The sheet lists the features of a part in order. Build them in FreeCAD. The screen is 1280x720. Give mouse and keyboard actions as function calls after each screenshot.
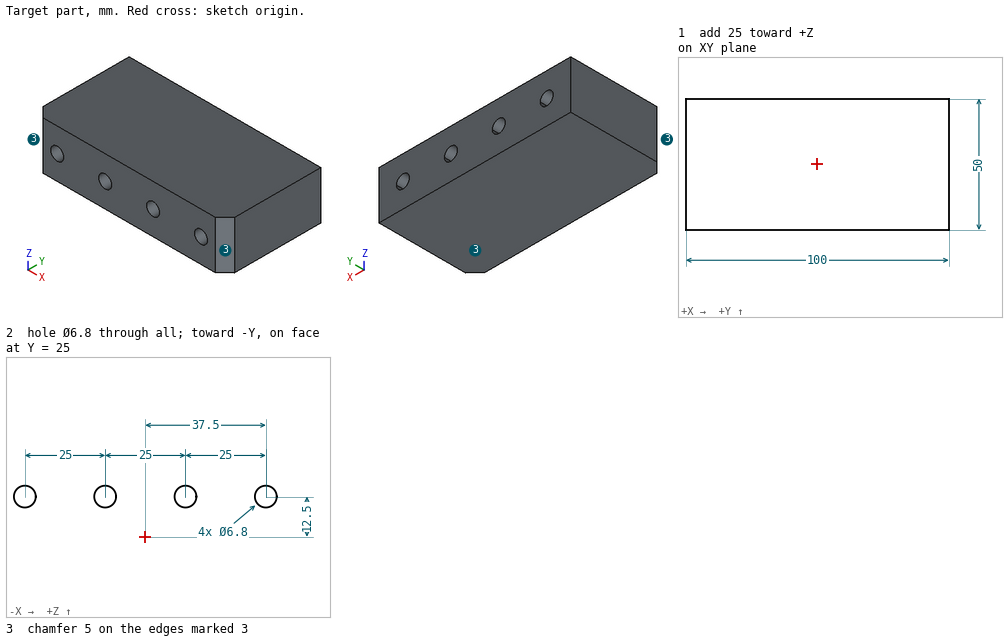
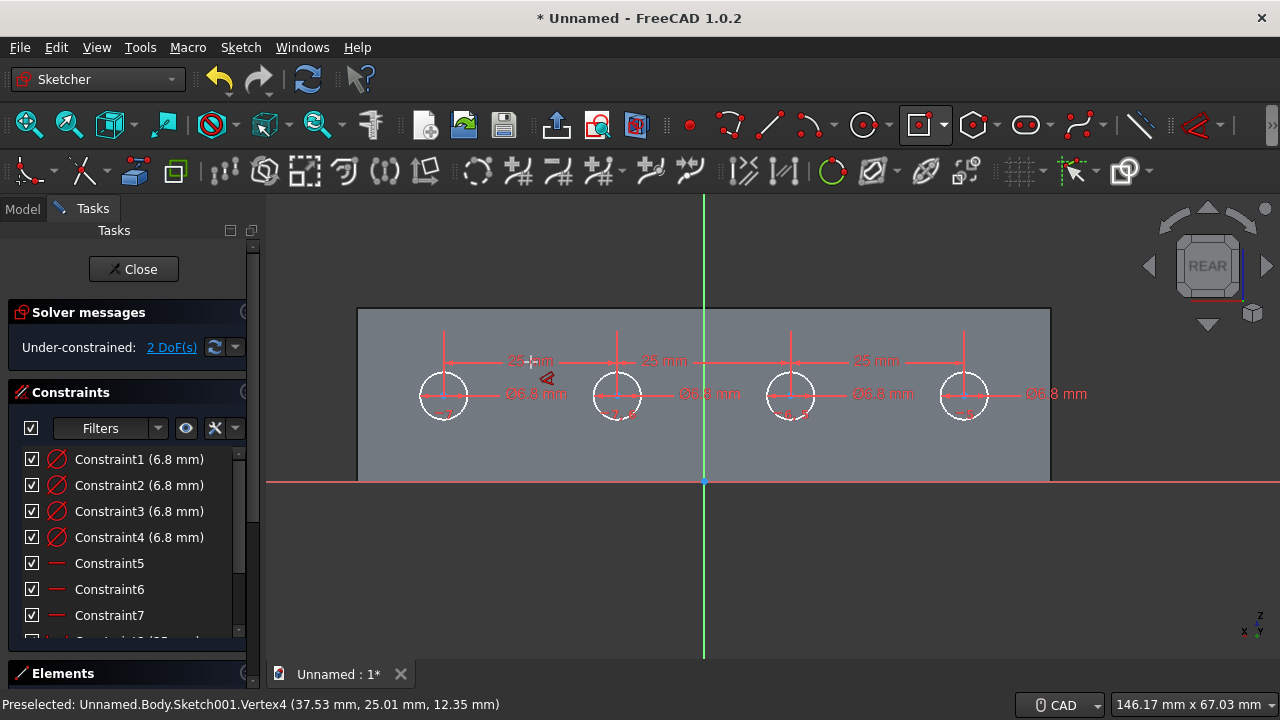
click(964, 396)
click(834, 516)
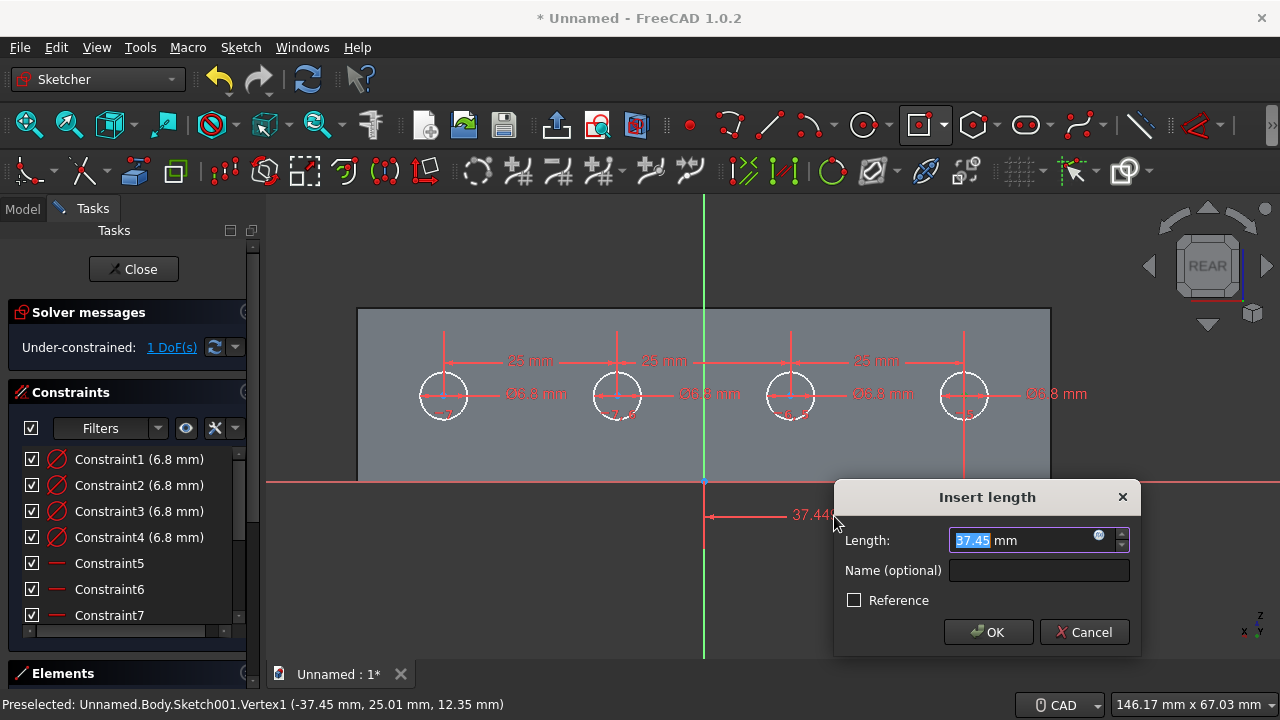
text(37.5)
key(Return)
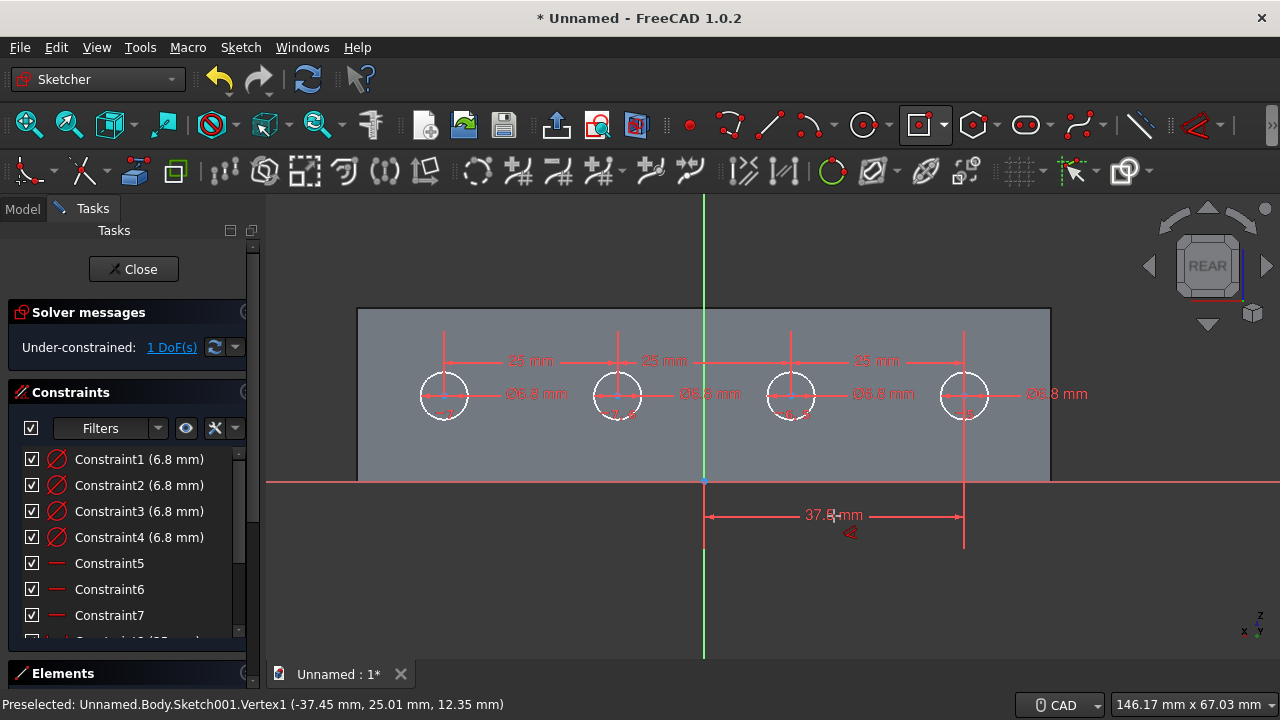
click(964, 396)
click(998, 439)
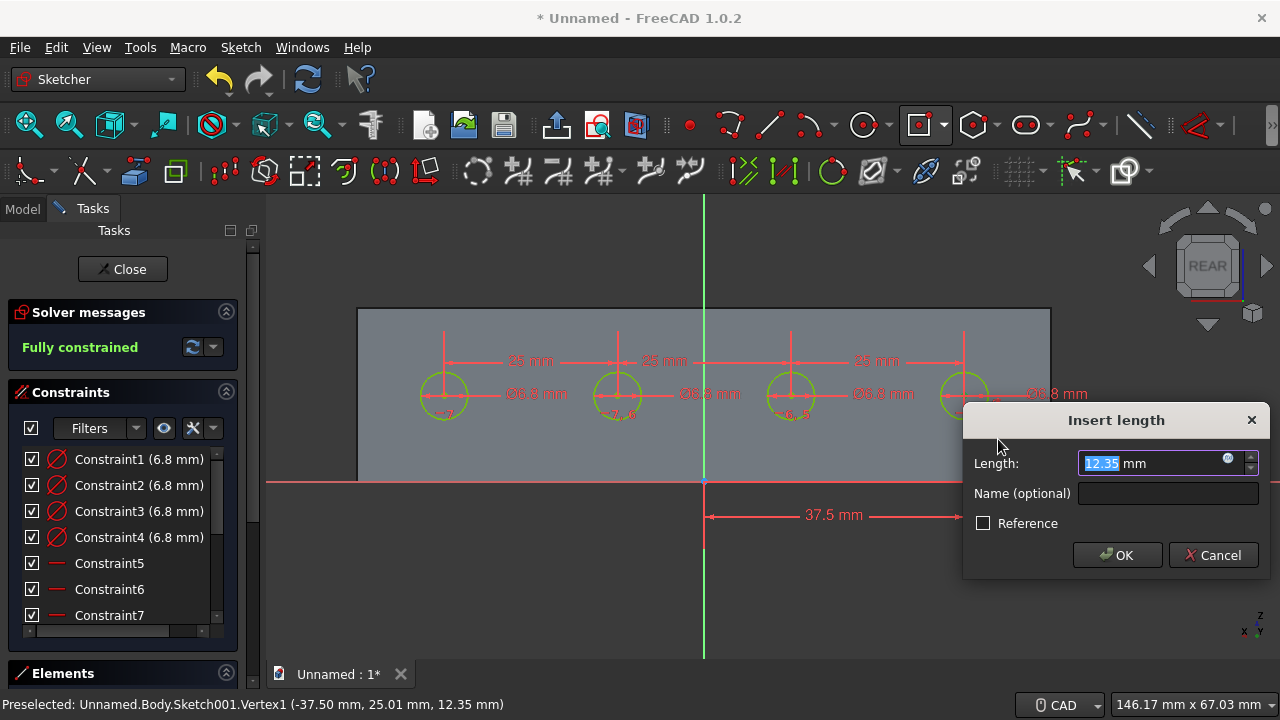
text(12.5)
key(Return)
key(Escape)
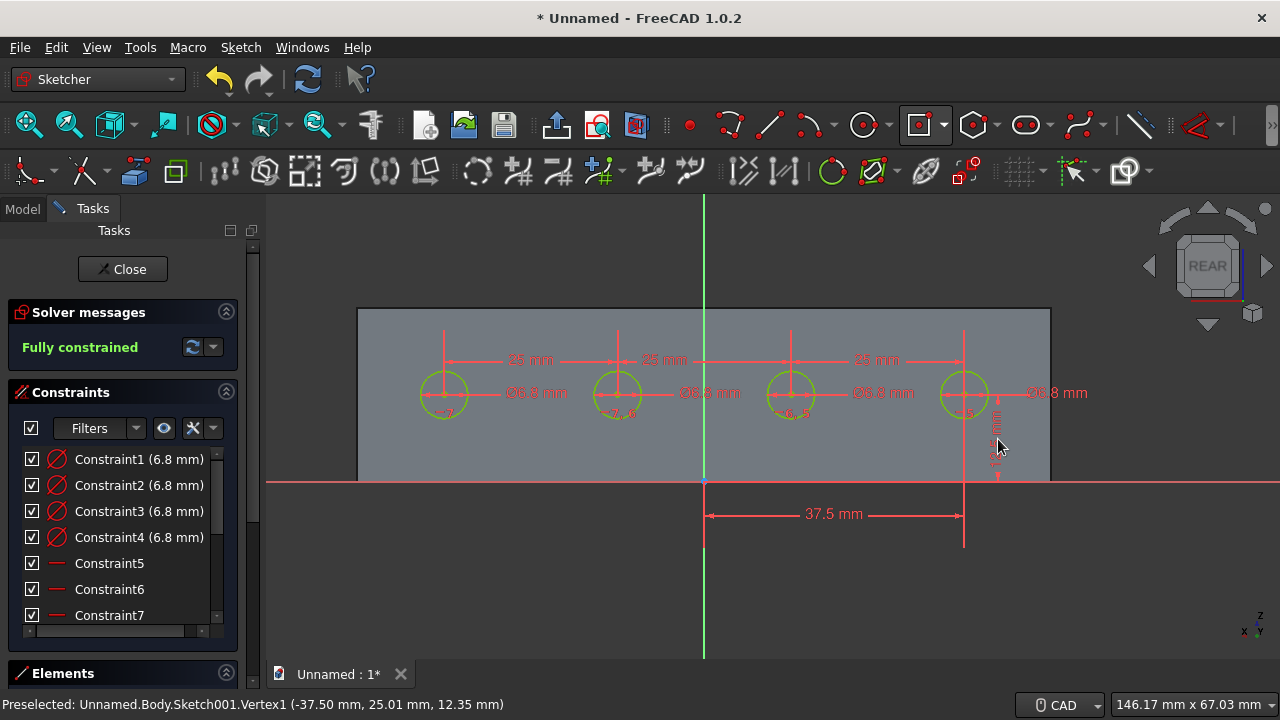
click(123, 269)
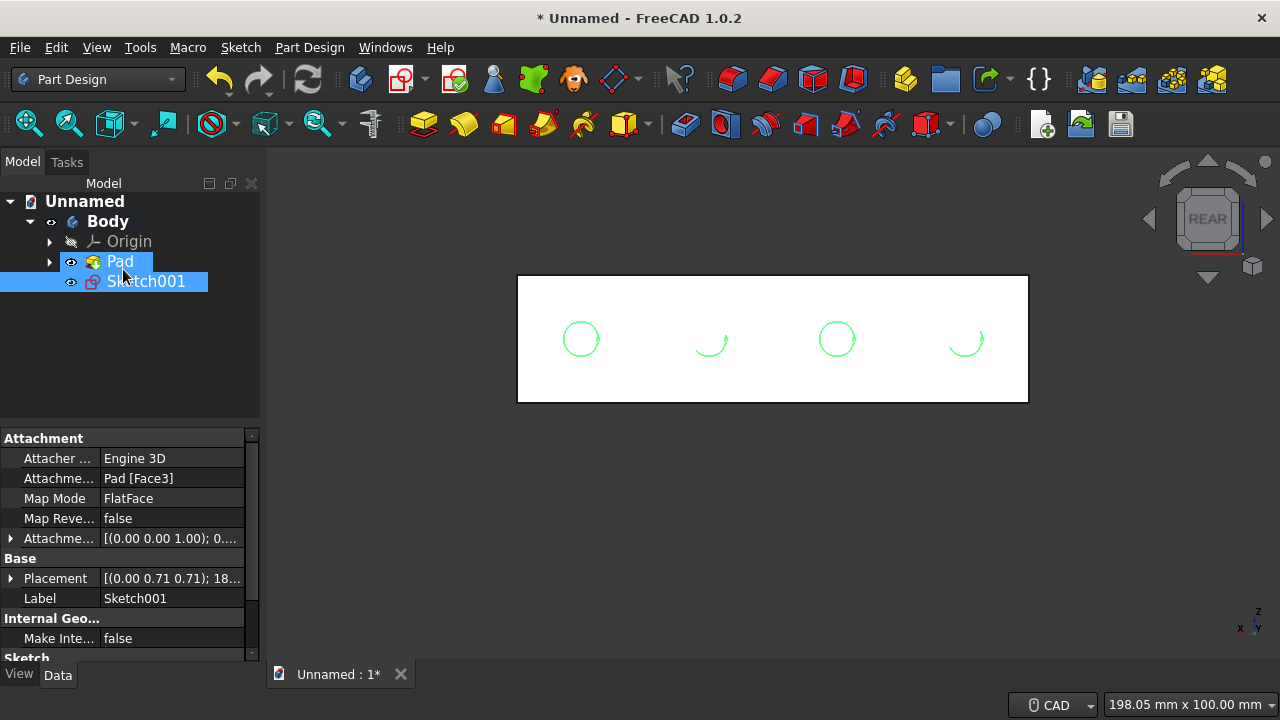
click(726, 124)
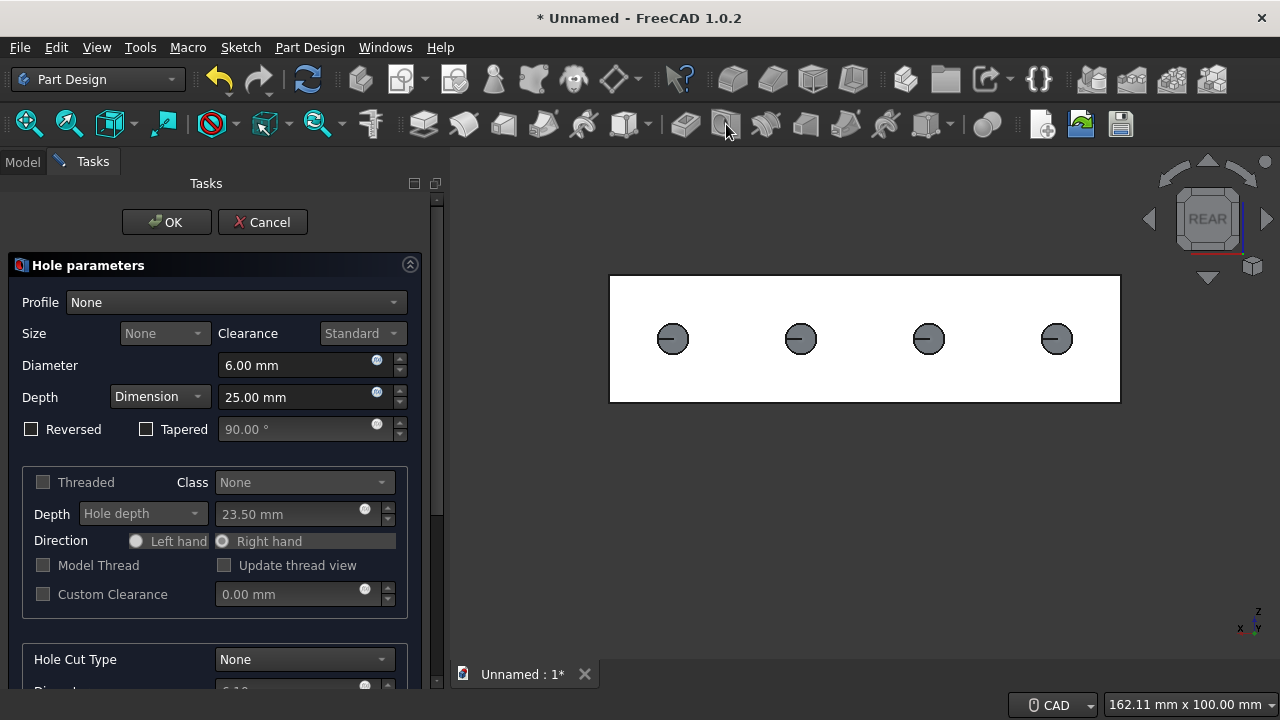
triple_click(305, 365)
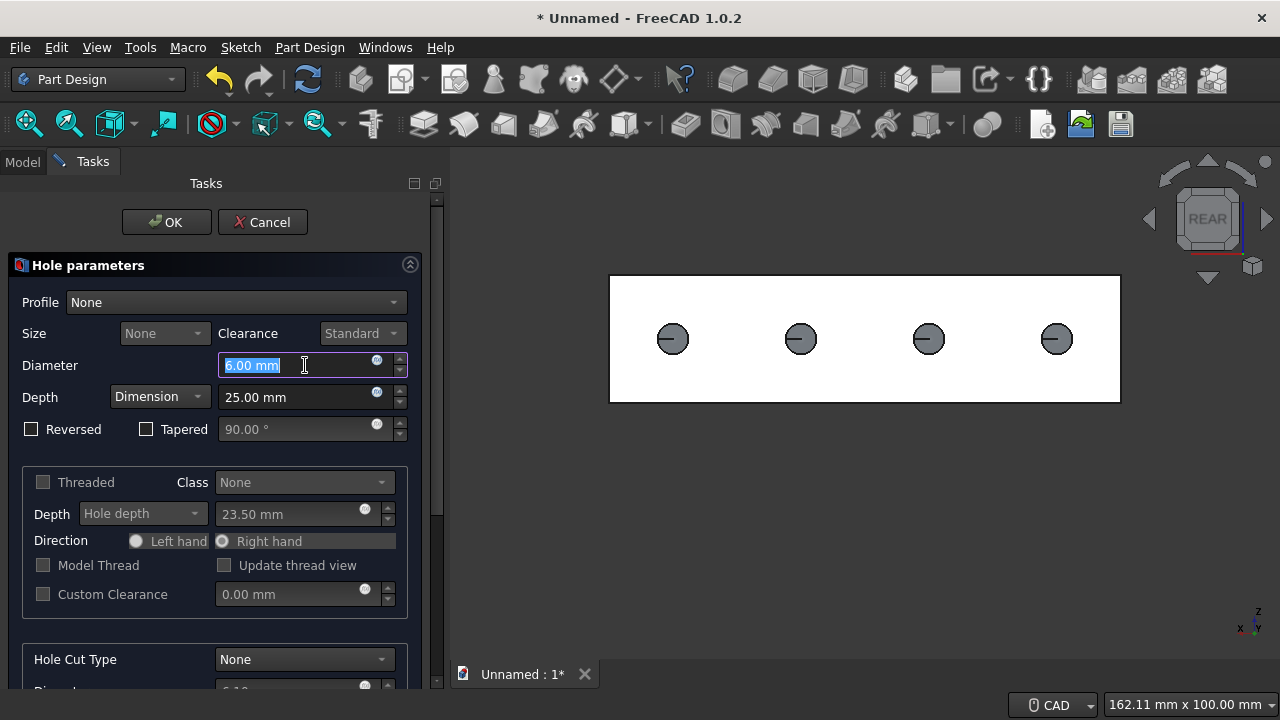
text(6.8)
key(Tab)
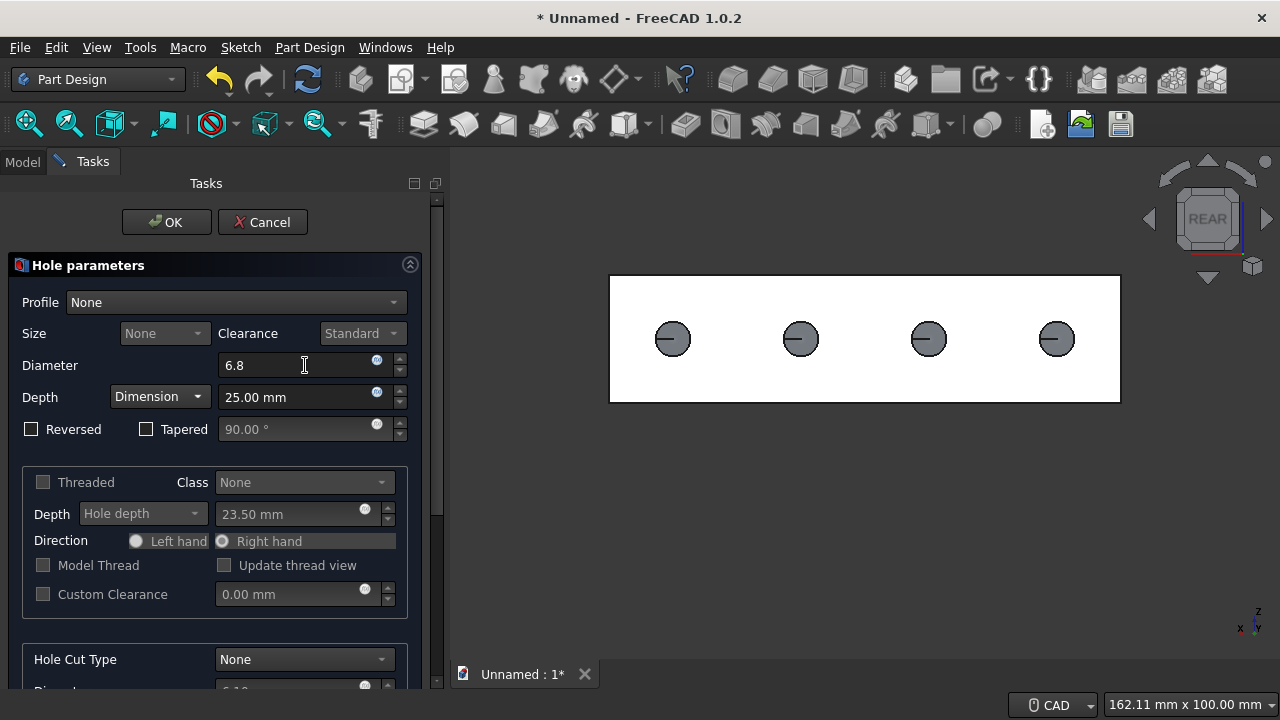
click(161, 396)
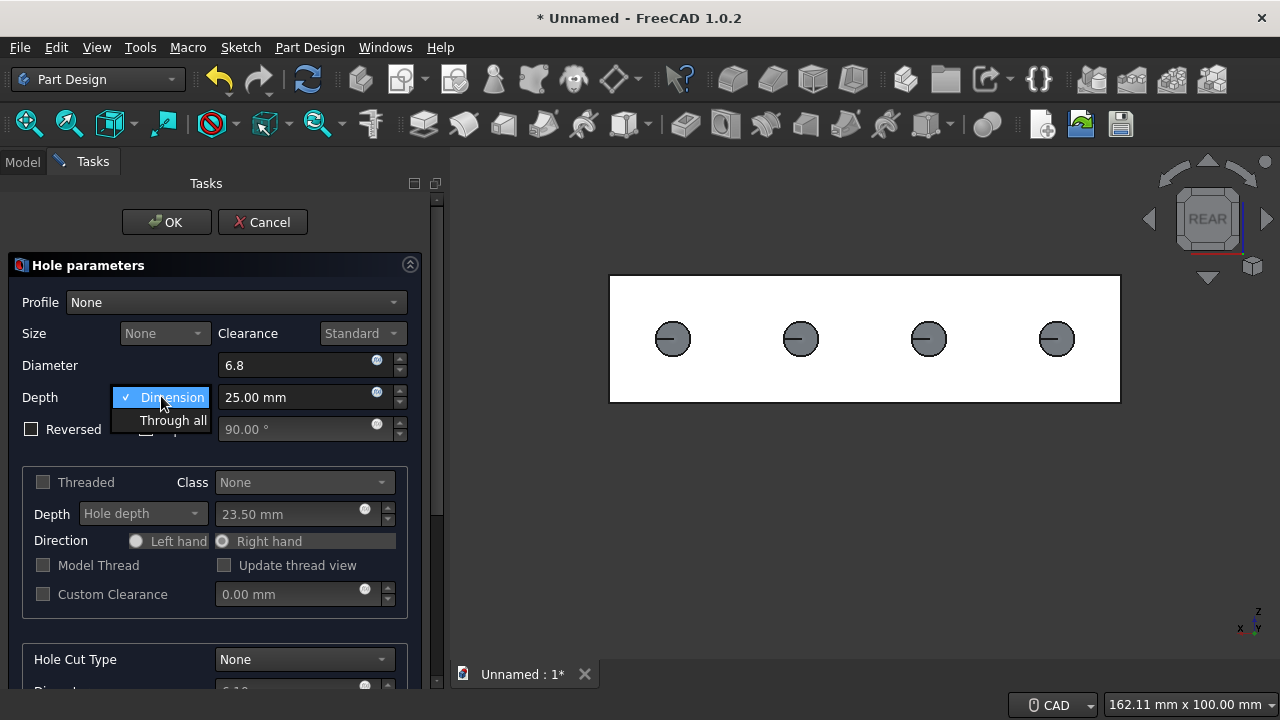
click(160, 420)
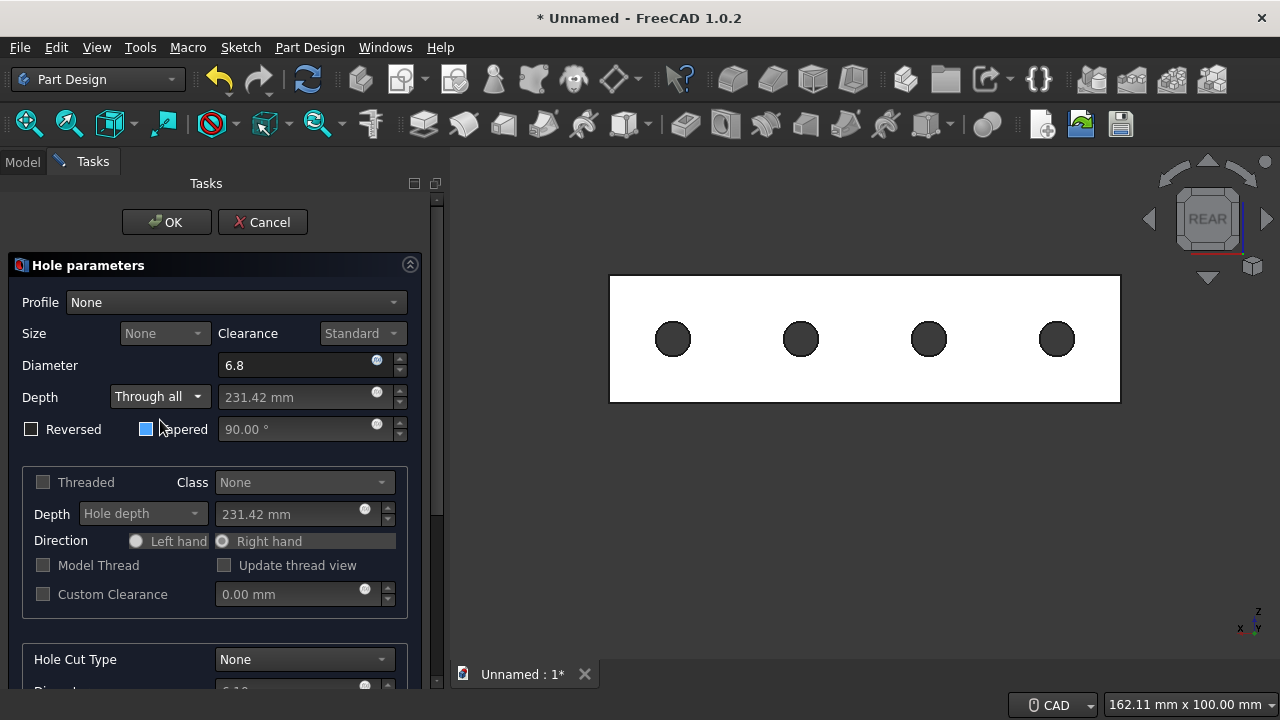
click(167, 222)